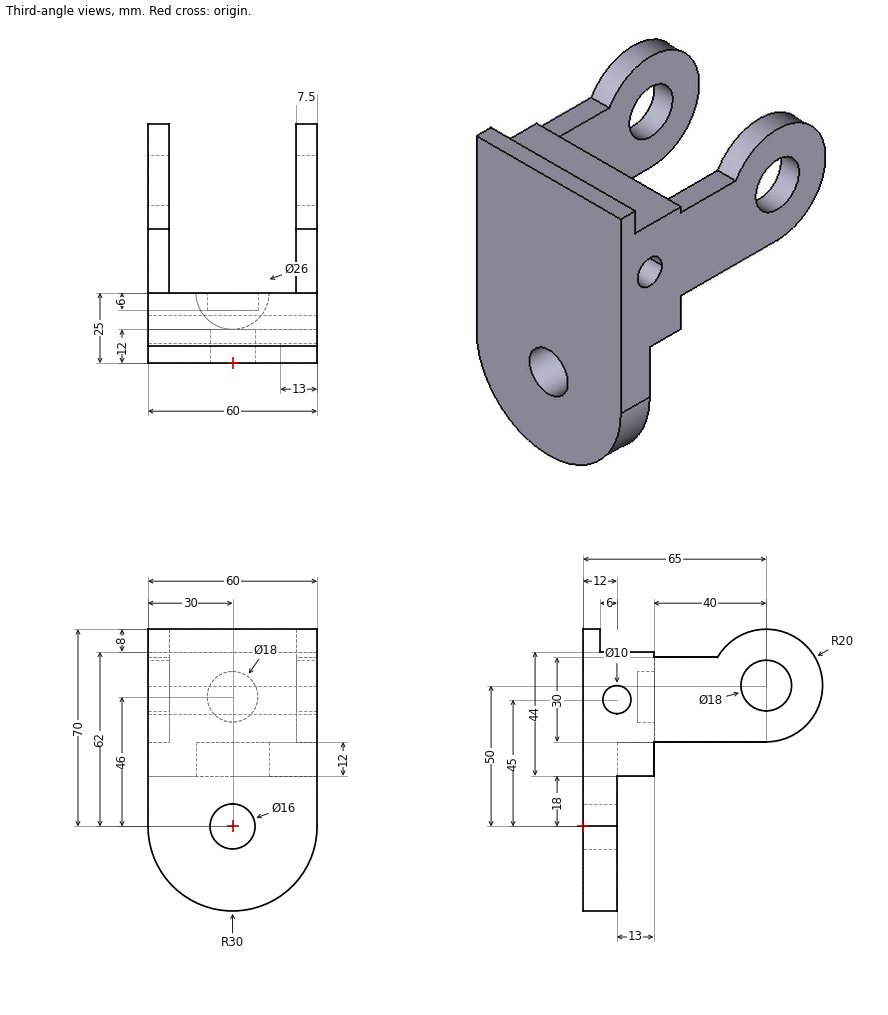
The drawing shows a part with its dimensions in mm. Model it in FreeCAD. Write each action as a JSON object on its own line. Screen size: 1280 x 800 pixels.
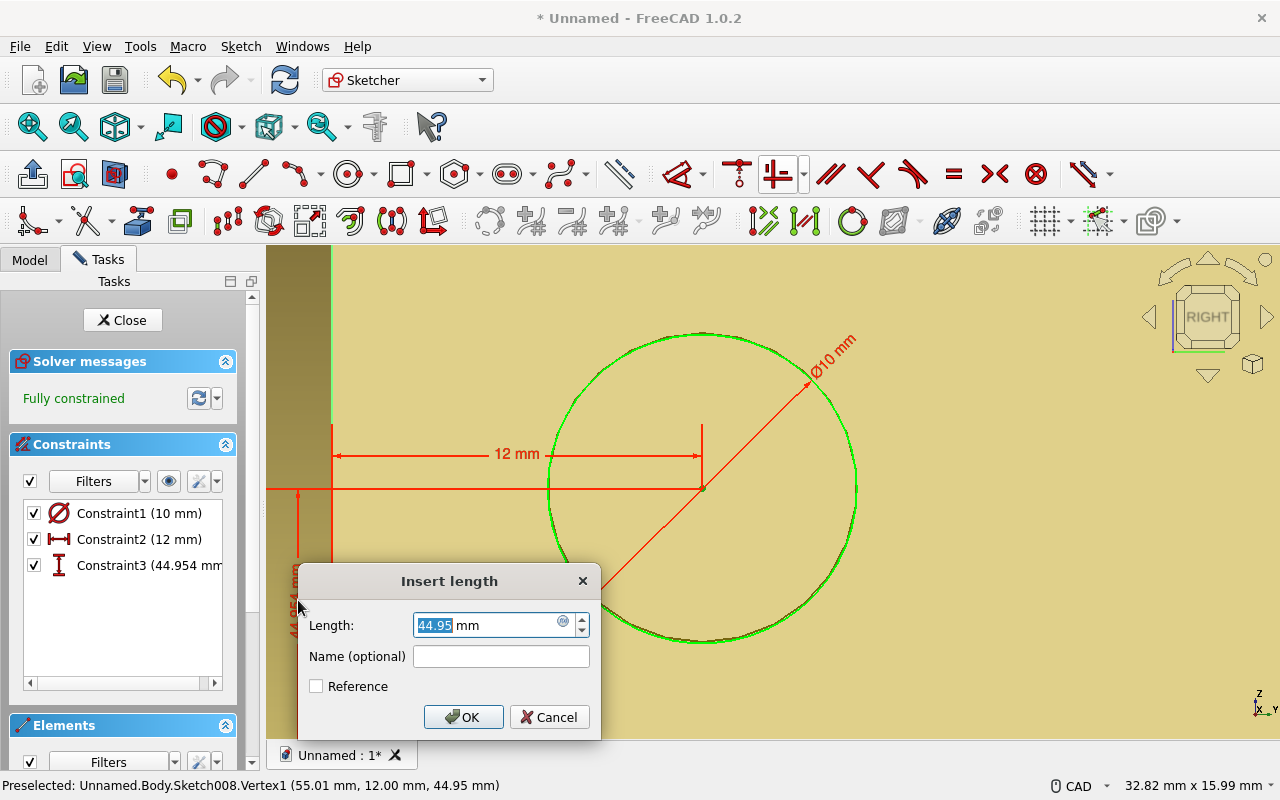
{"action": "type", "text": "45"}
{"action": "key", "text": "Return"}
{"action": "key", "text": "Escape"}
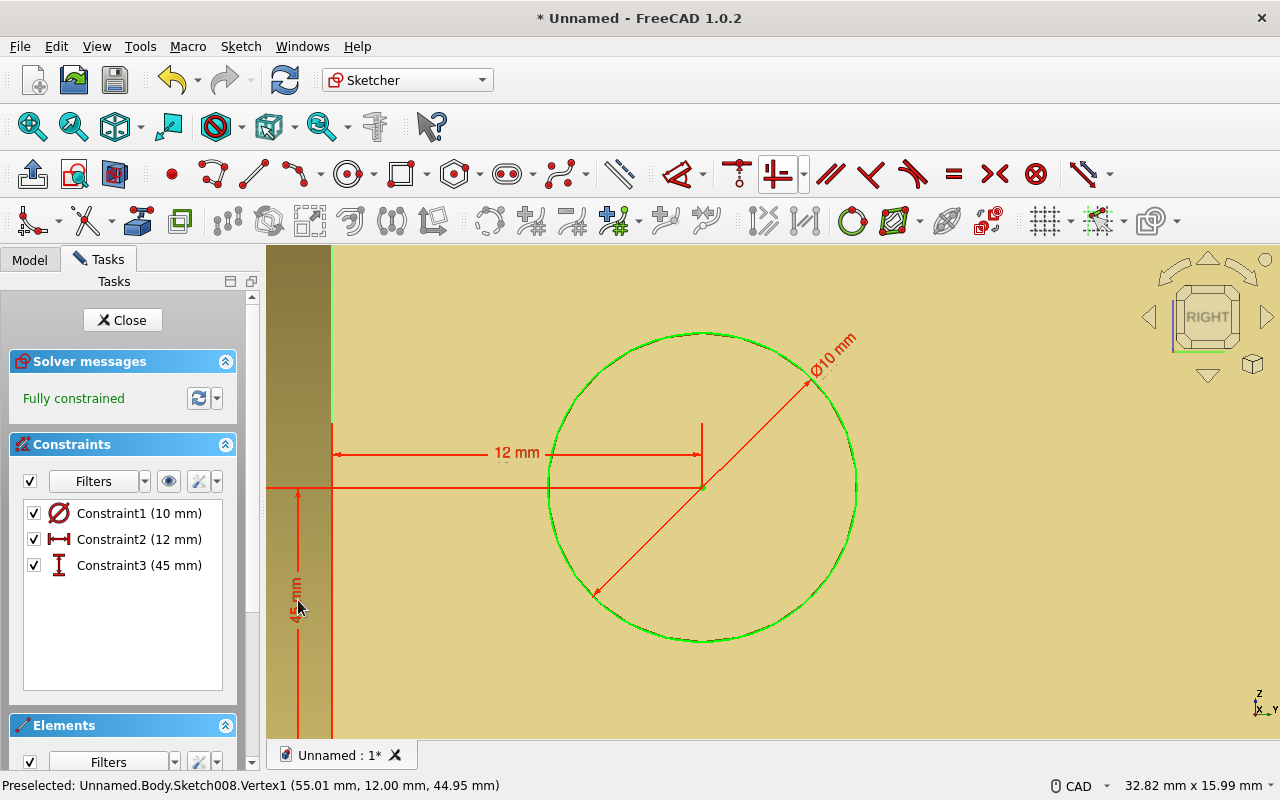
{"action": "left_click", "coordinate": [123, 320]}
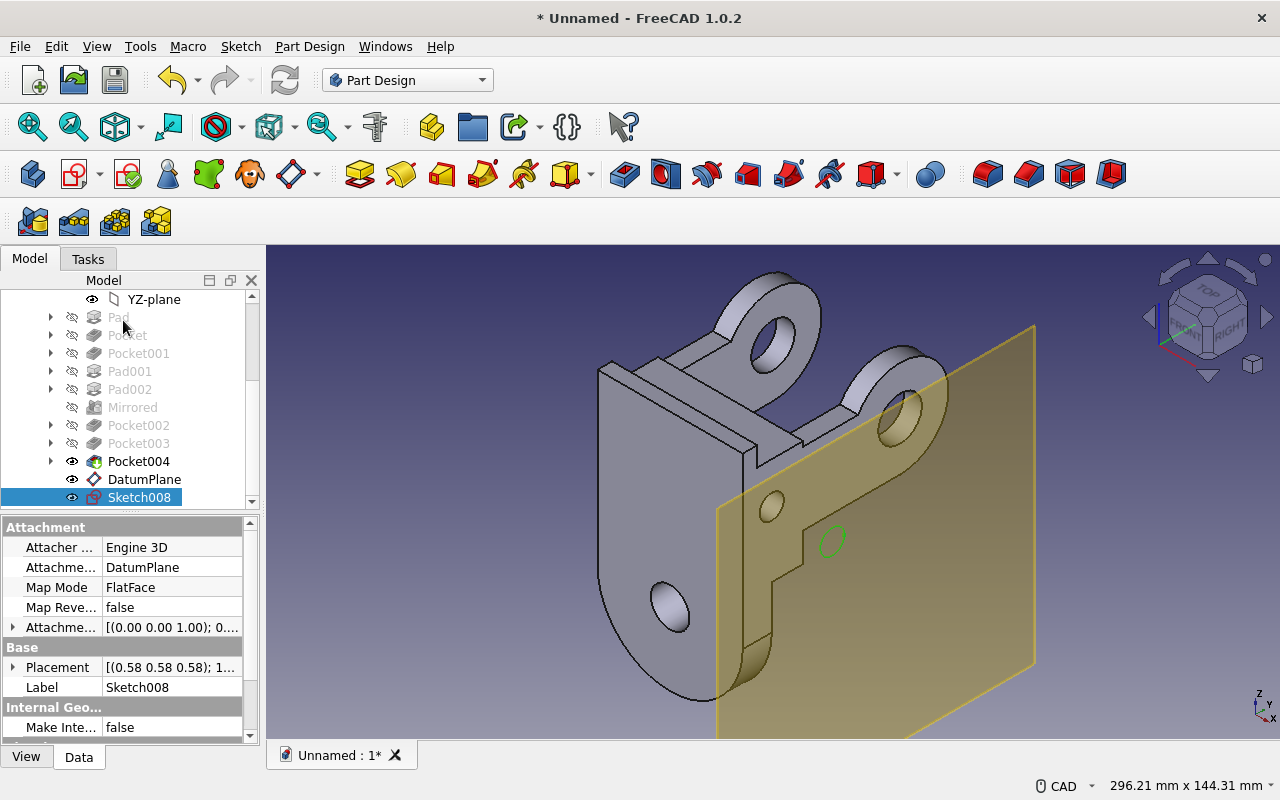
{"action": "left_click", "coordinate": [625, 174]}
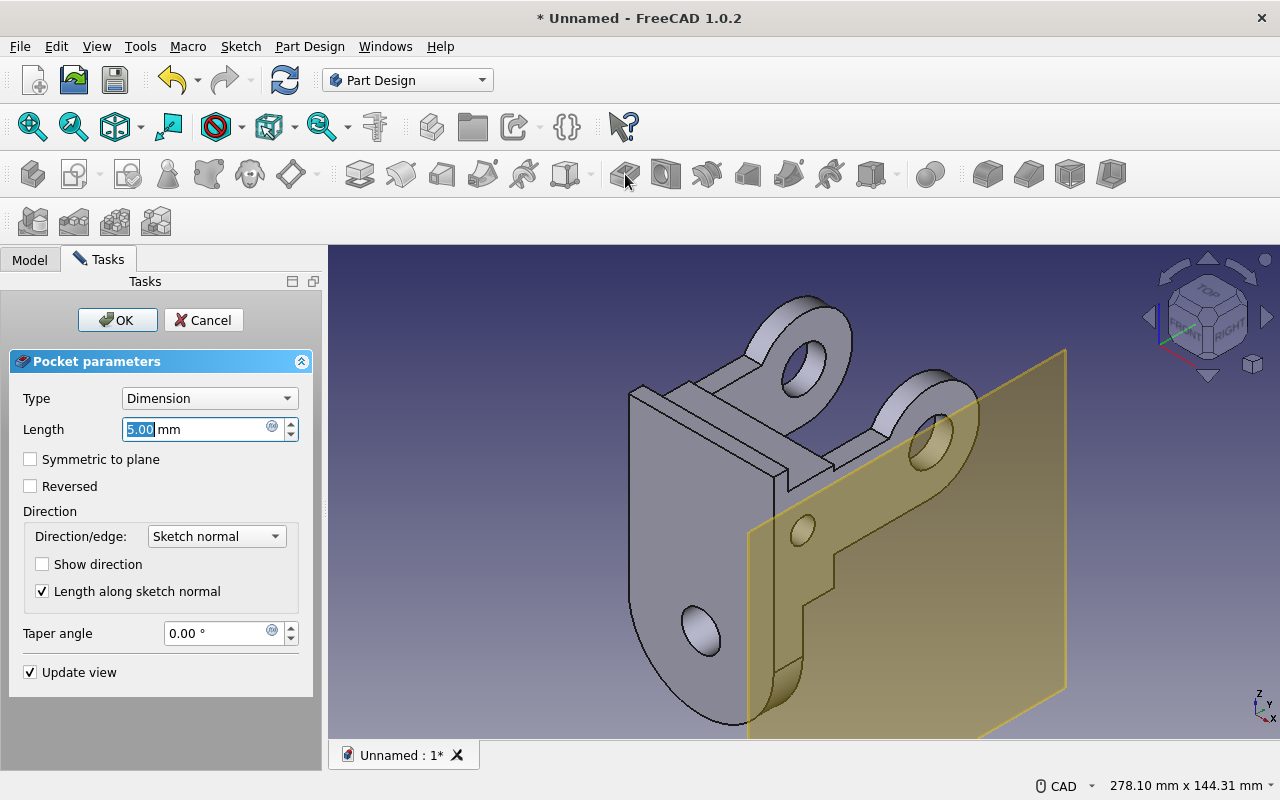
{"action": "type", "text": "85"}
{"action": "key", "text": "Tab"}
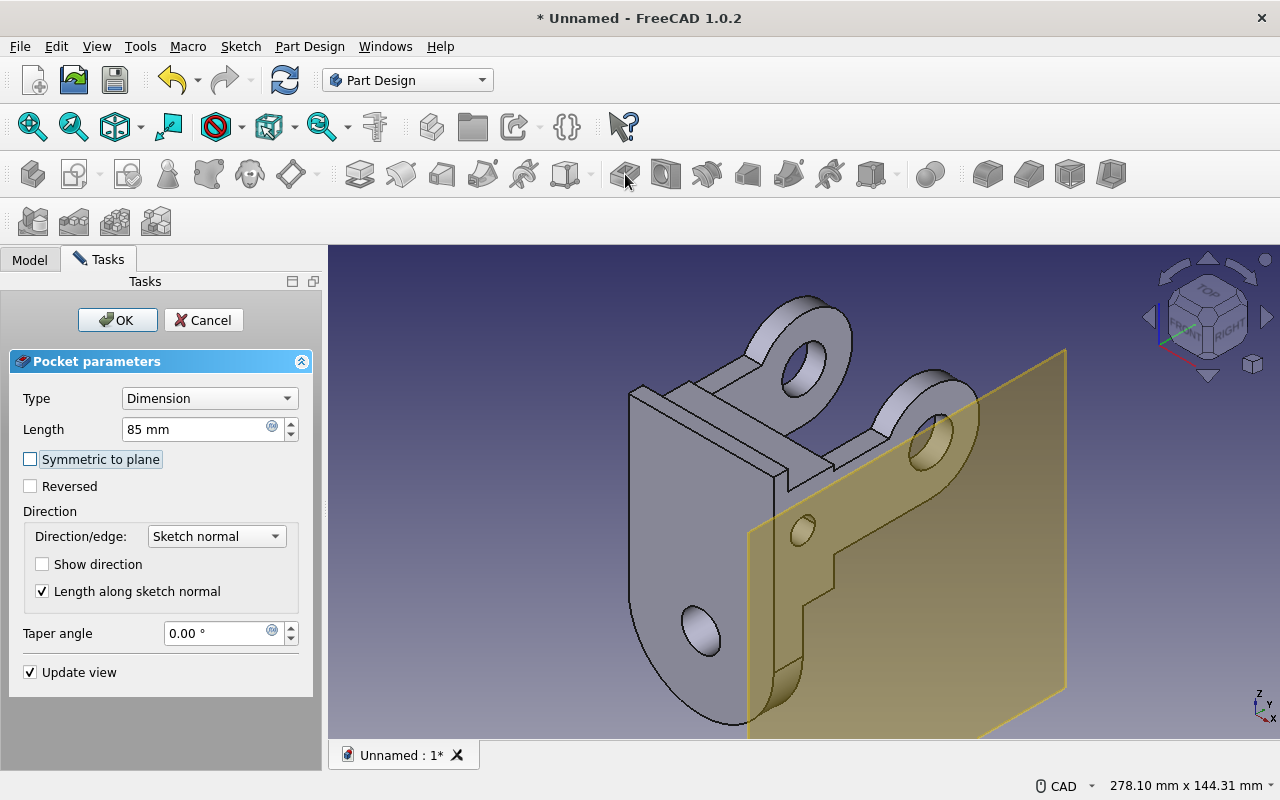
{"action": "left_click", "coordinate": [118, 320]}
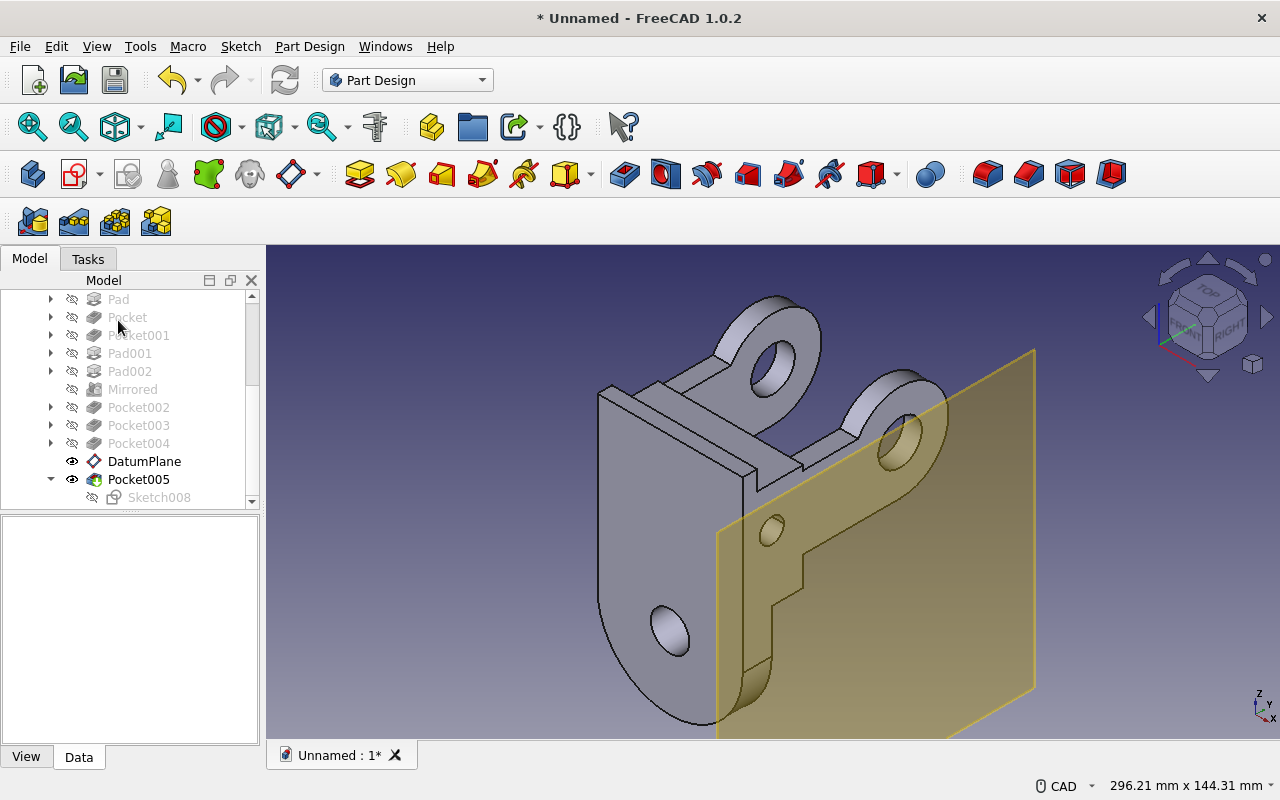
{"action": "left_click", "coordinate": [117, 461]}
{"action": "key", "text": "space"}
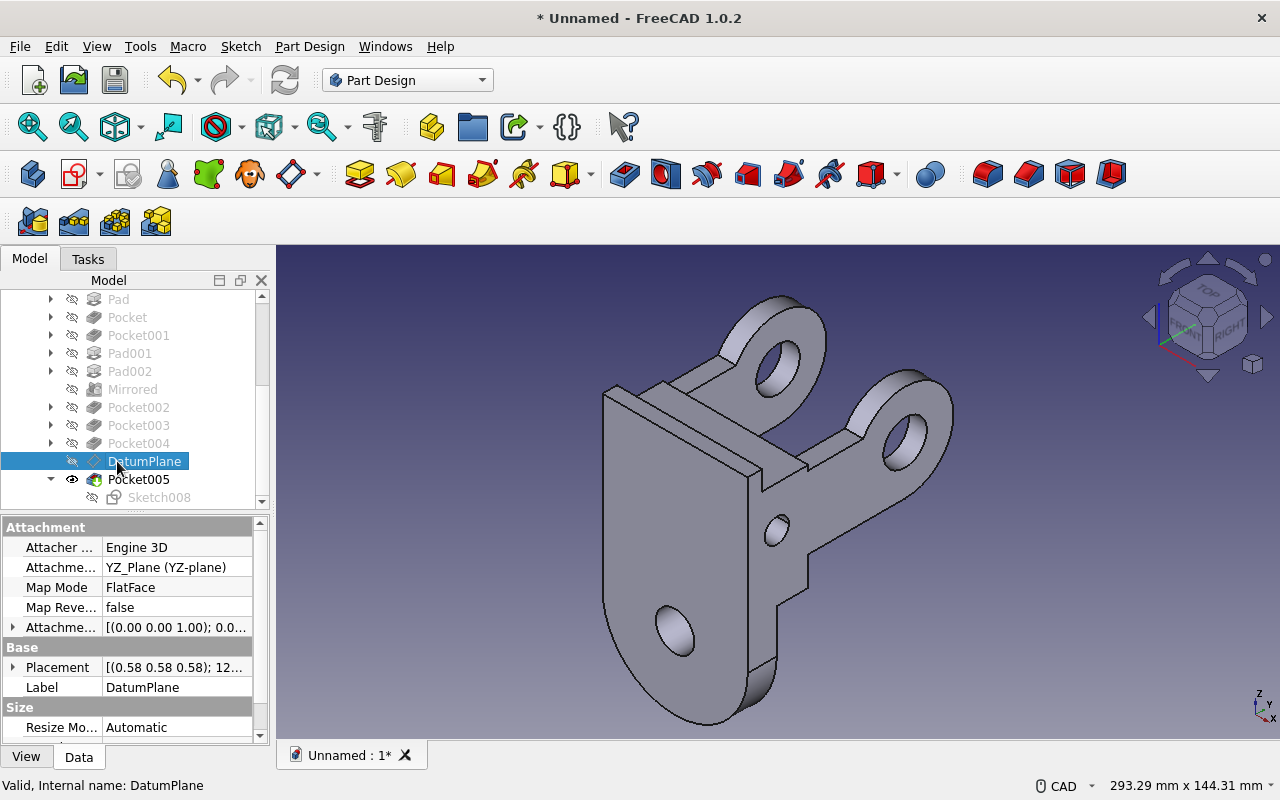
{"action": "key", "text": "v f"}